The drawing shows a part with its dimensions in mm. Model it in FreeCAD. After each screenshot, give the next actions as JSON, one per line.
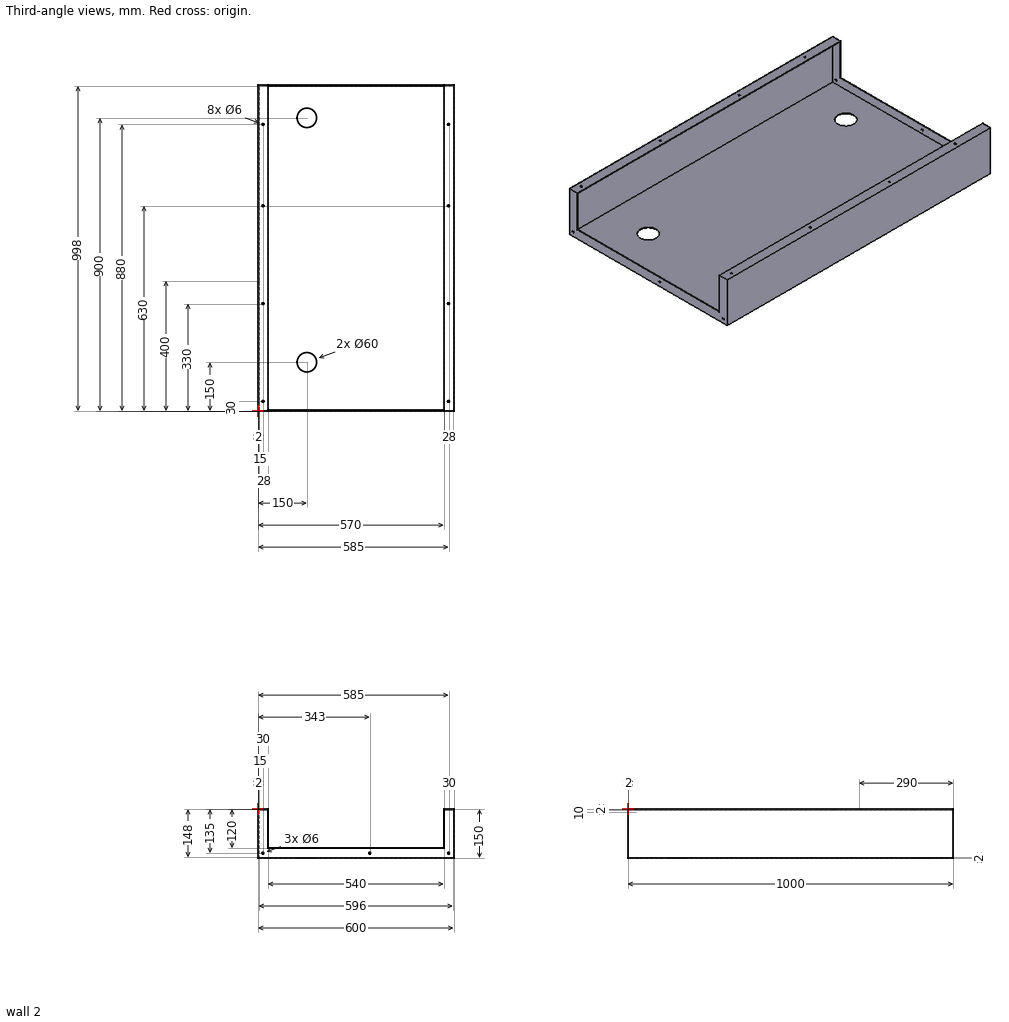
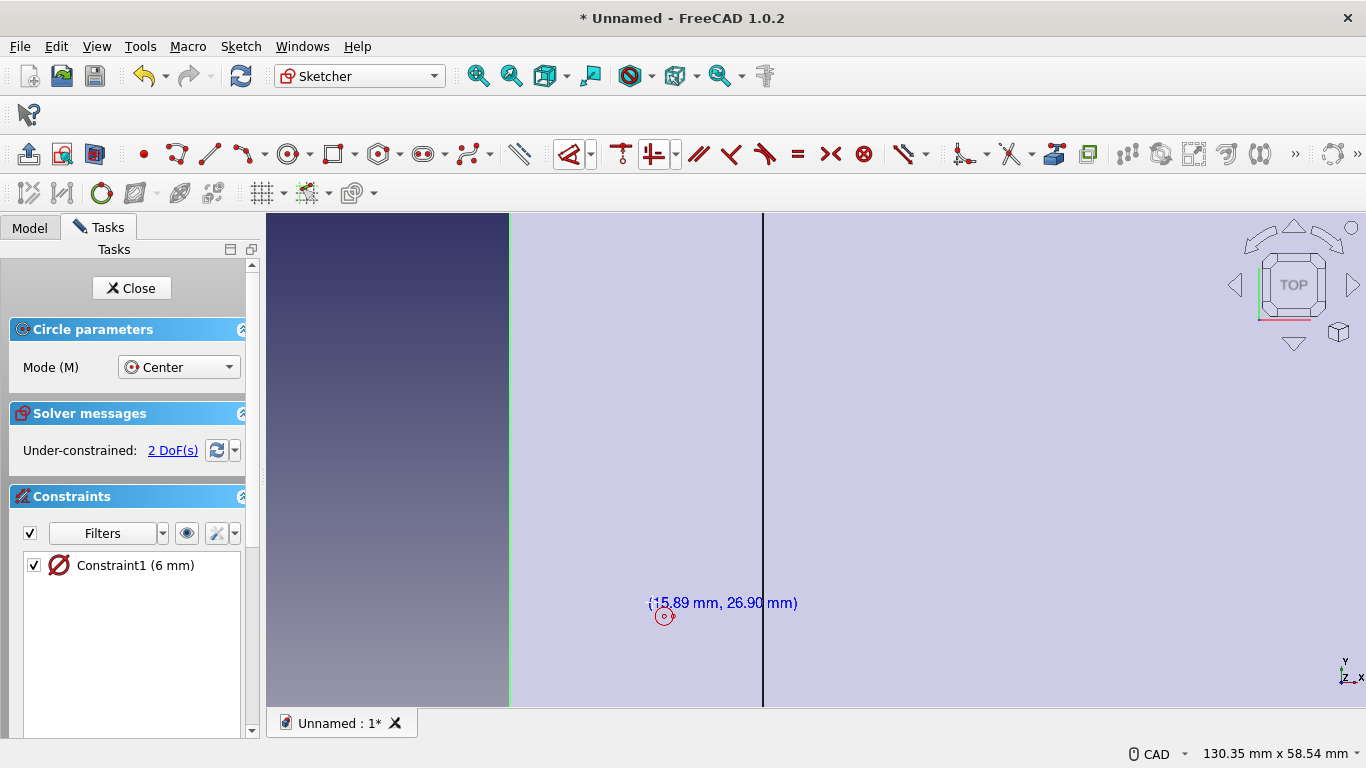
{"action": "scroll", "coordinate": [630, 636], "scroll_direction": "down", "scroll_amount": 15}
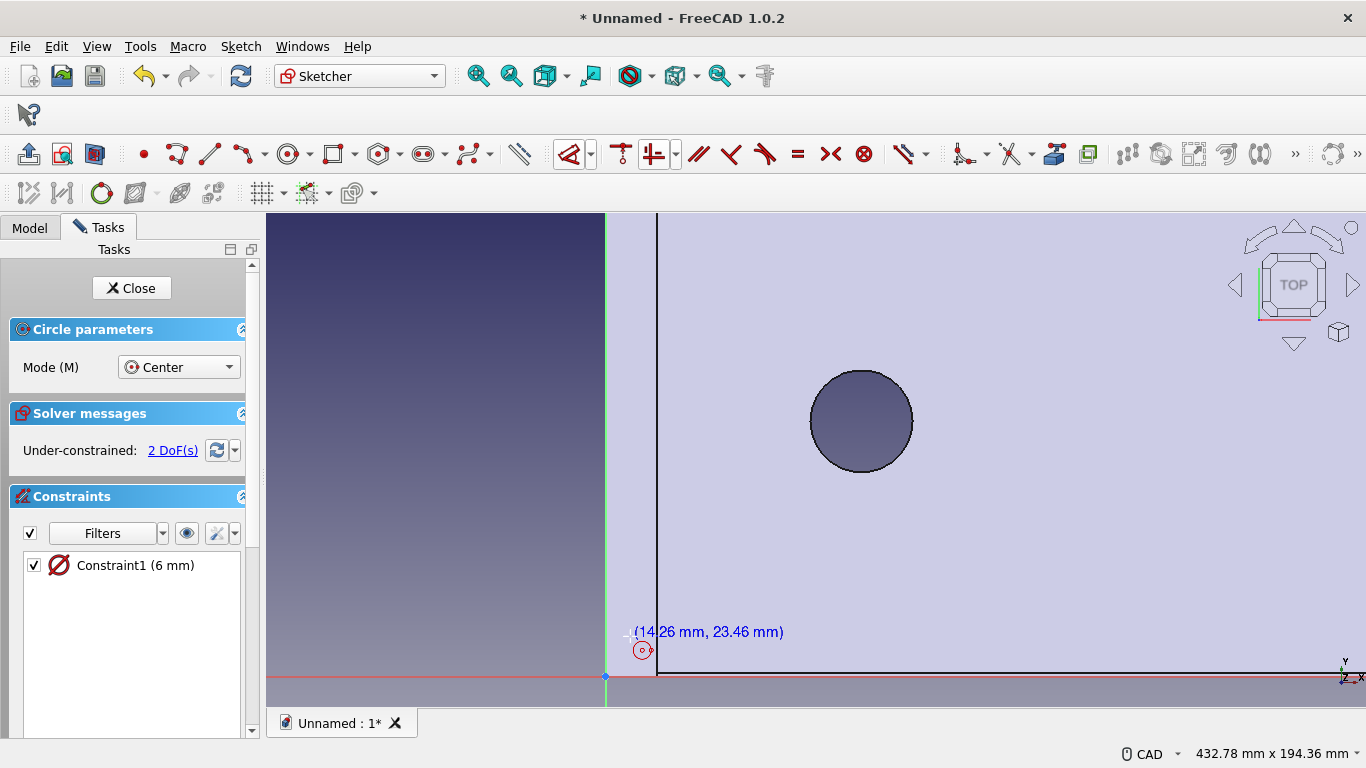
{"action": "scroll", "coordinate": [631, 634], "scroll_direction": "up", "scroll_amount": 5}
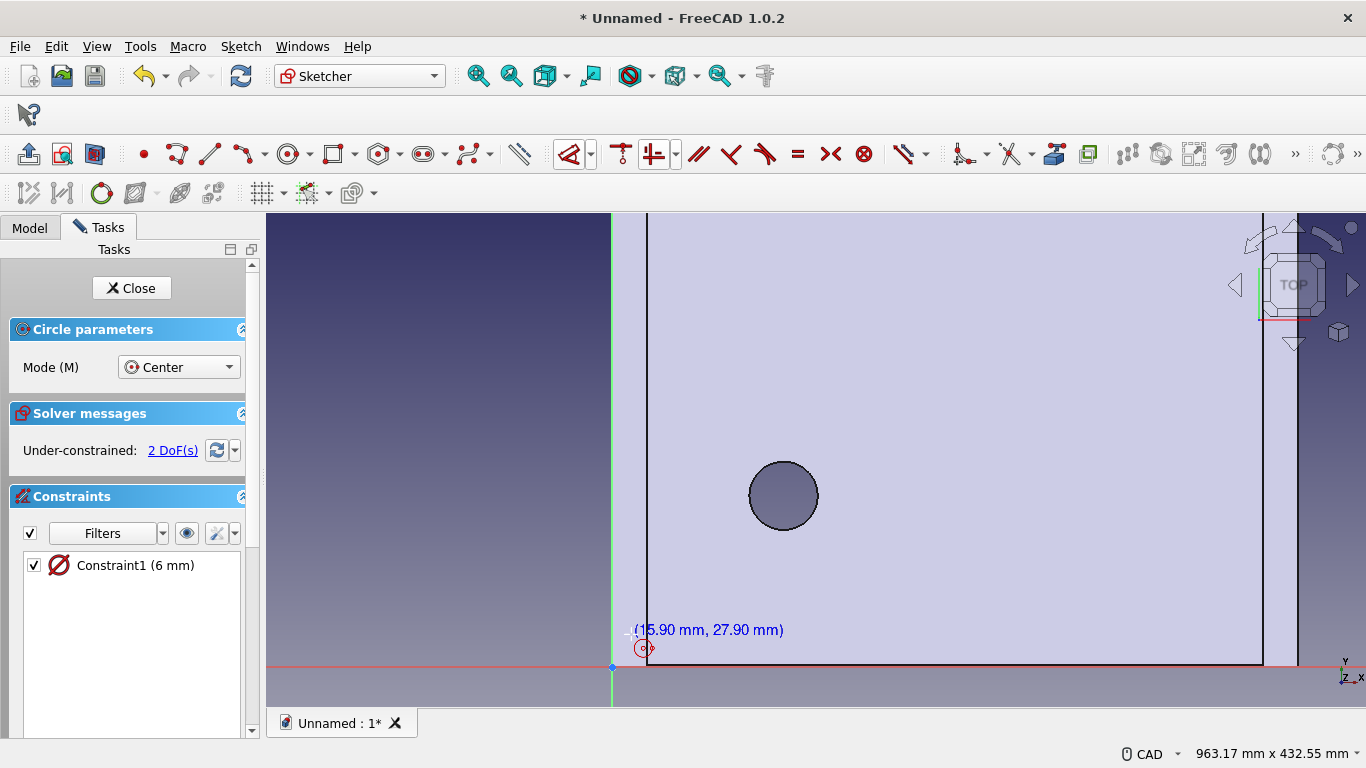
{"action": "left_click", "coordinate": [629, 633]}
{"action": "mouse_move", "coordinate": [632, 630]}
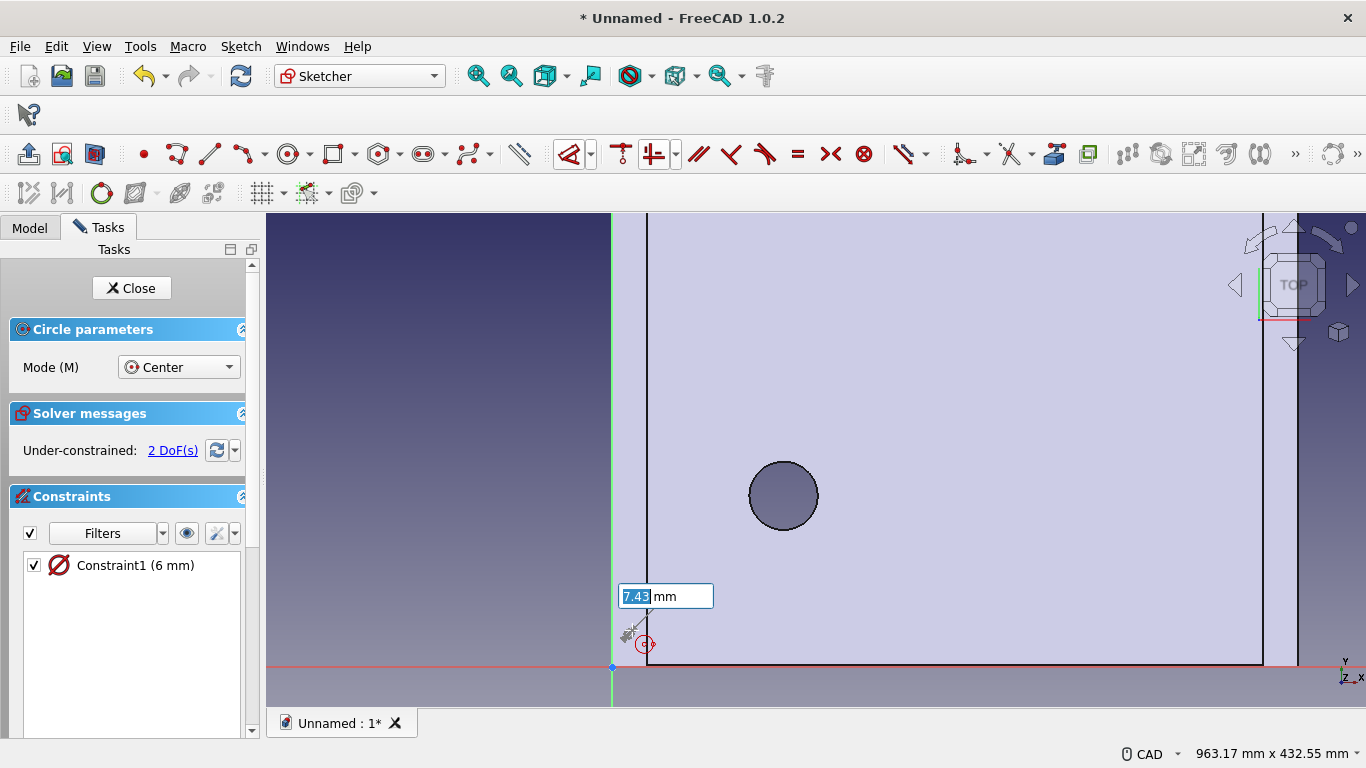
{"action": "type", "text": "6"}
{"action": "key", "text": "Return"}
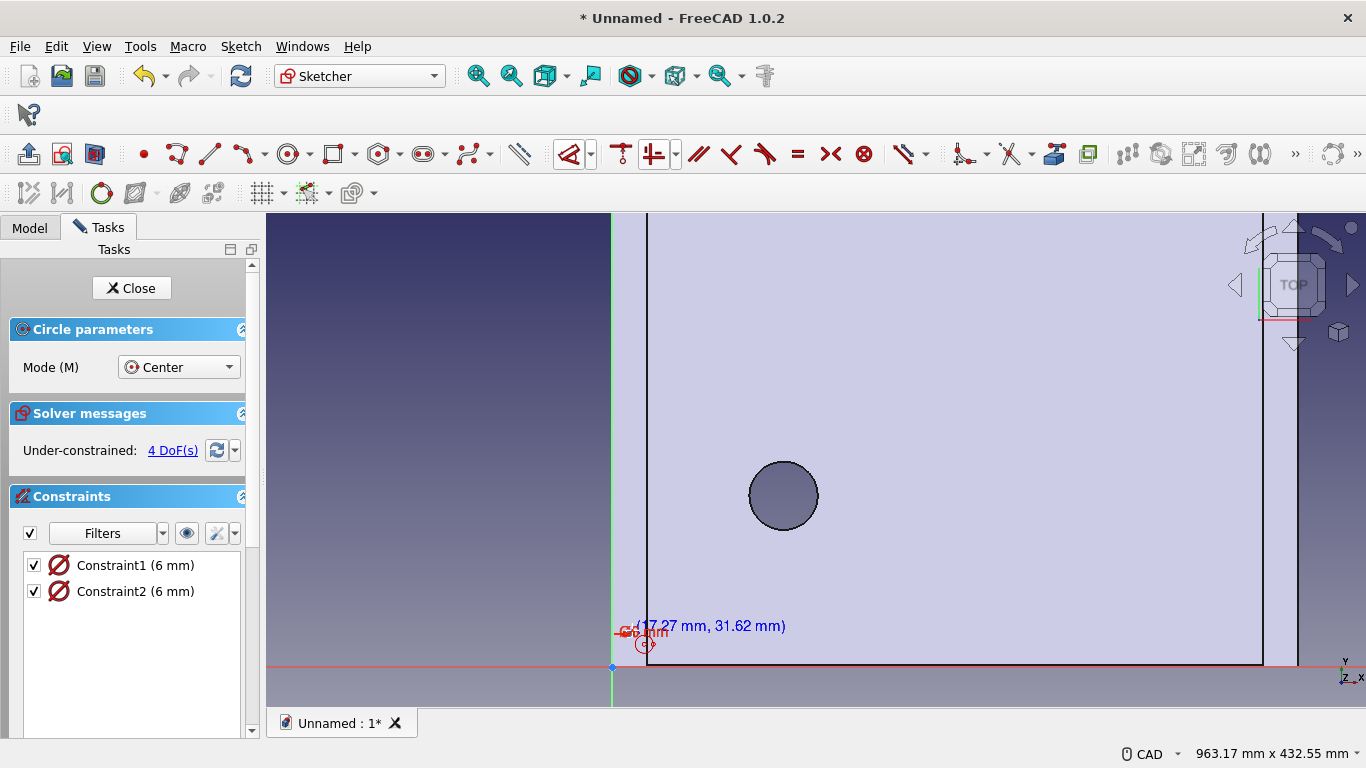
{"action": "scroll", "coordinate": [661, 588], "scroll_direction": "down", "scroll_amount": 6}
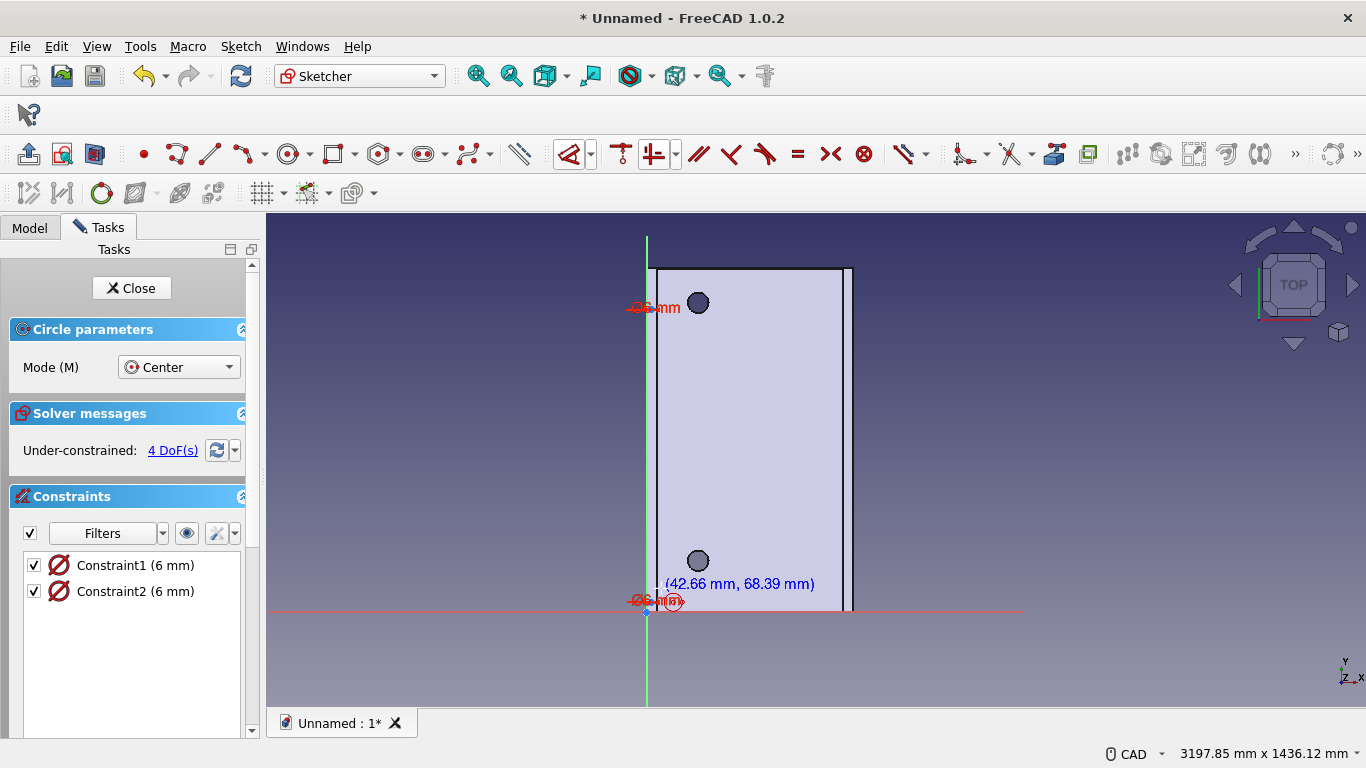
{"action": "scroll", "coordinate": [848, 310], "scroll_direction": "up", "scroll_amount": 16}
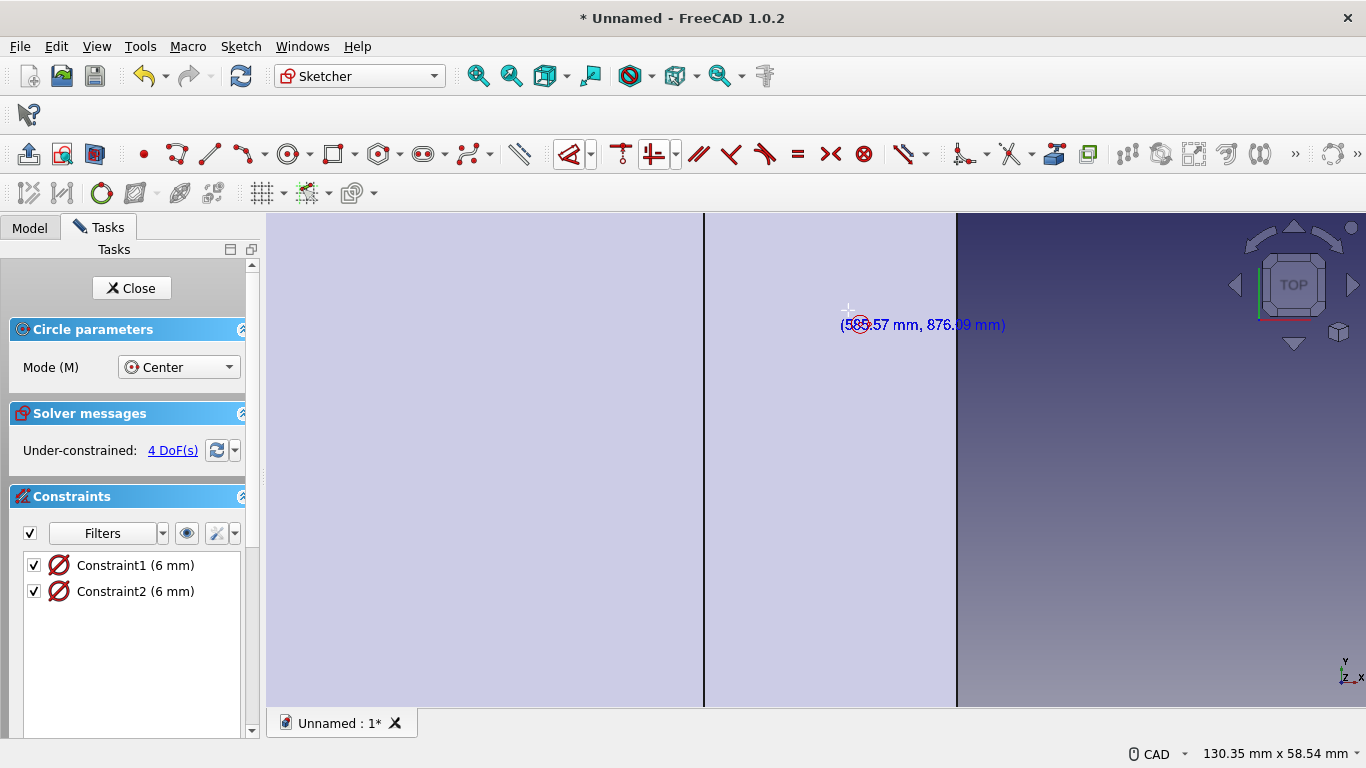
{"action": "scroll", "coordinate": [872, 275], "scroll_direction": "down", "scroll_amount": 15}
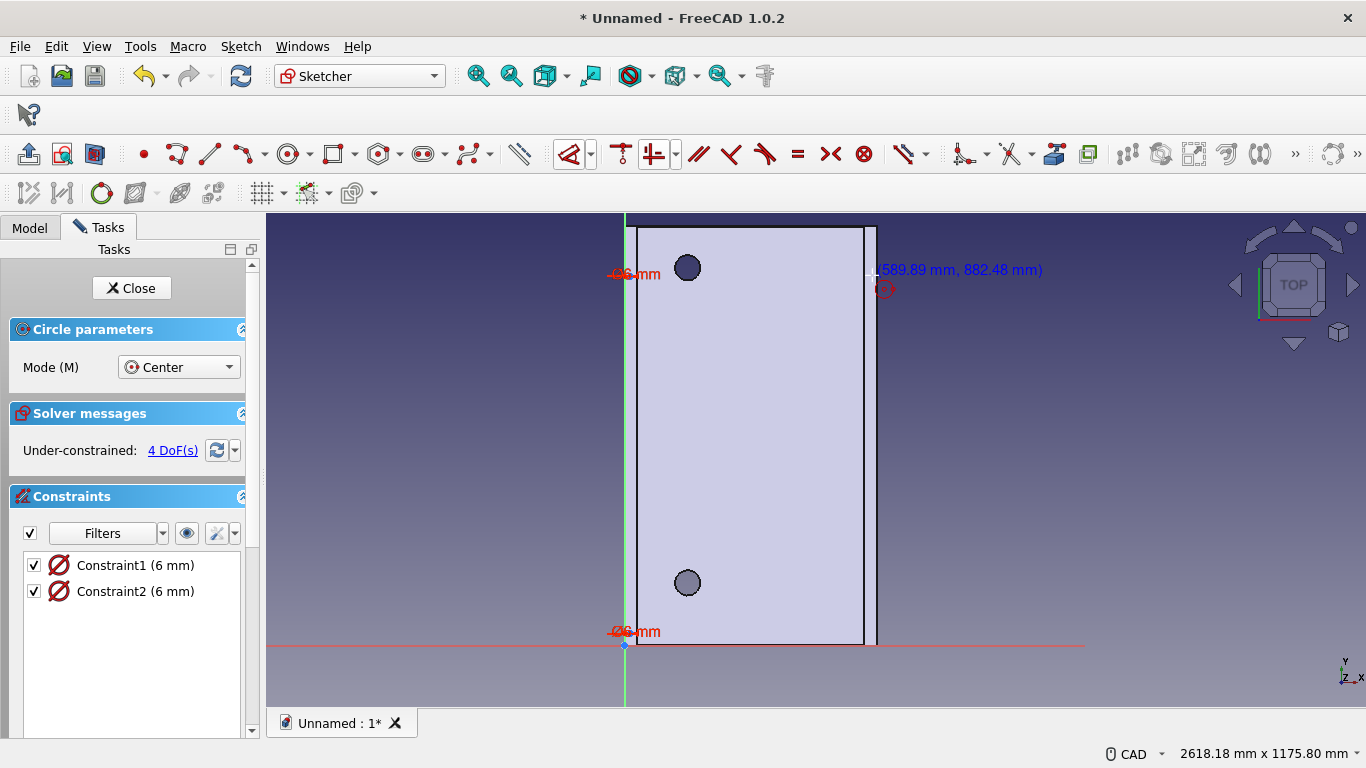
{"action": "left_click", "coordinate": [870, 276]}
{"action": "mouse_move", "coordinate": [871, 275]}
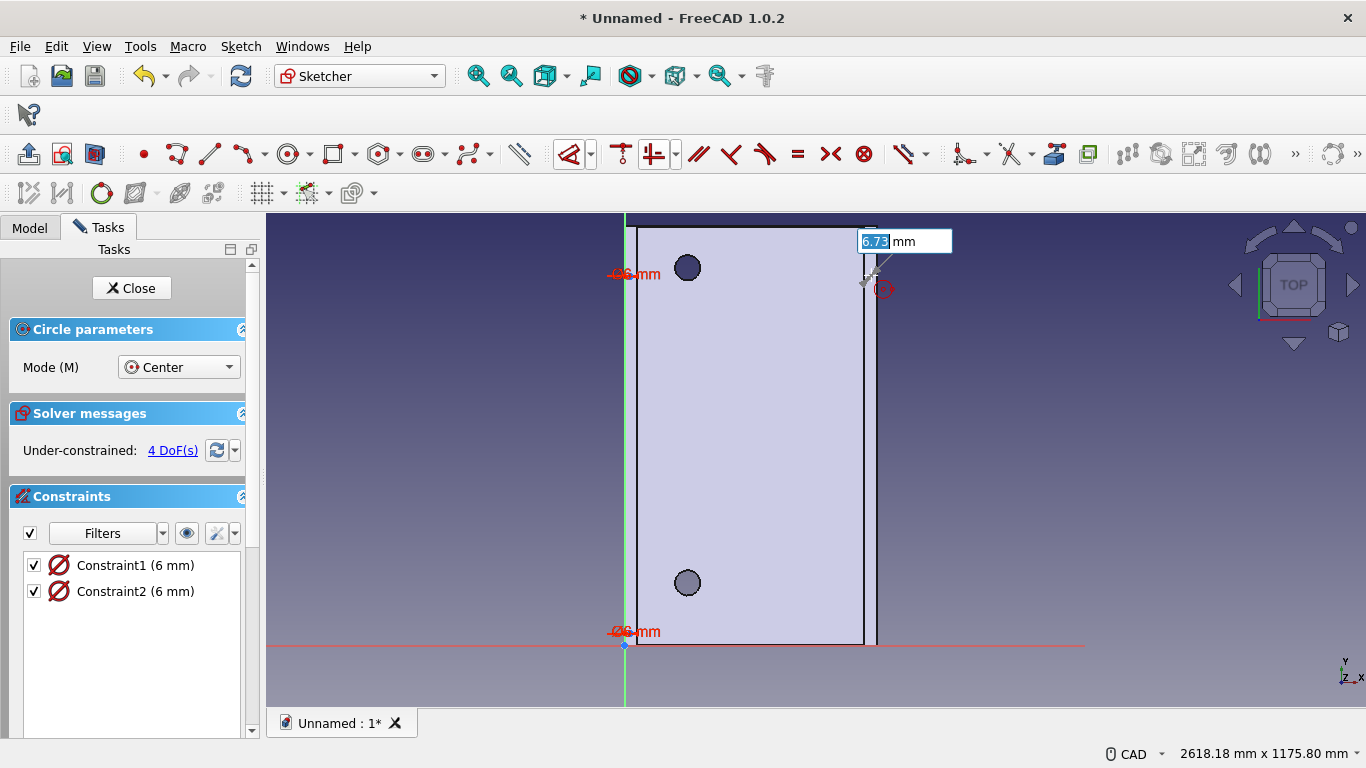
{"action": "type", "text": "6"}
{"action": "key", "text": "Return"}